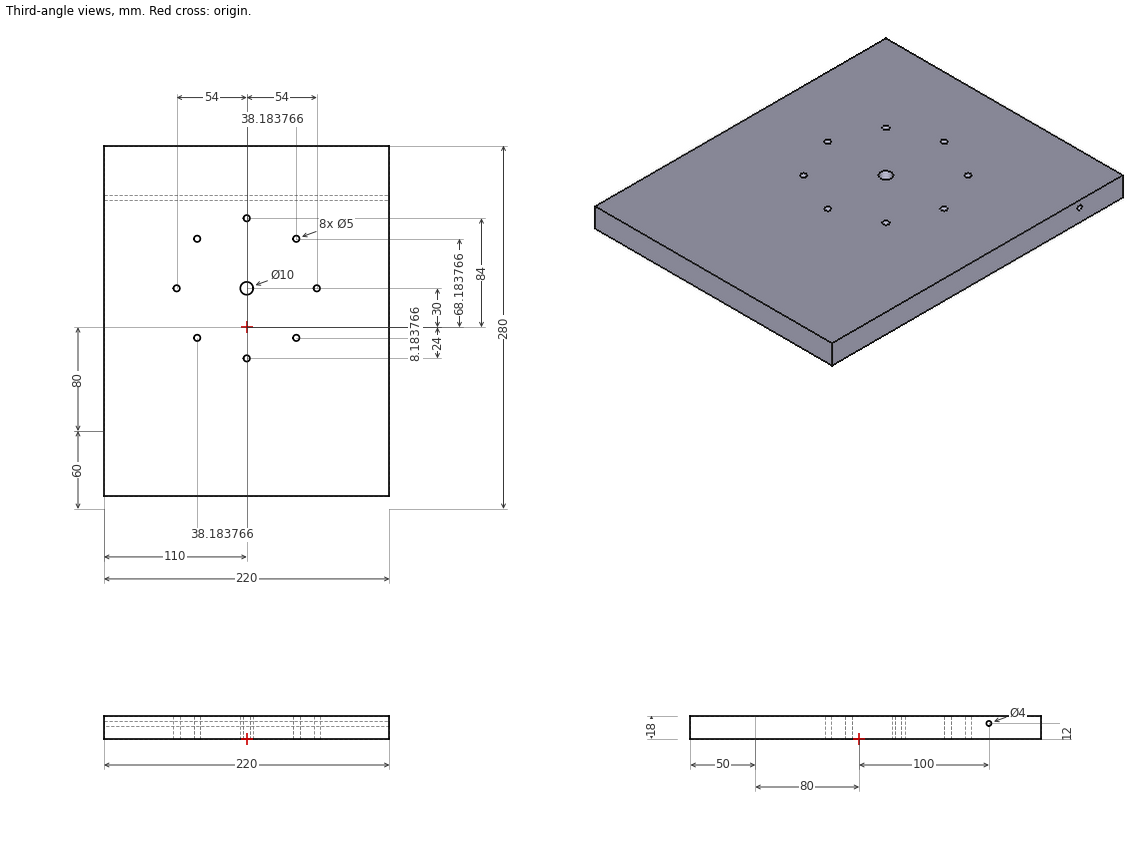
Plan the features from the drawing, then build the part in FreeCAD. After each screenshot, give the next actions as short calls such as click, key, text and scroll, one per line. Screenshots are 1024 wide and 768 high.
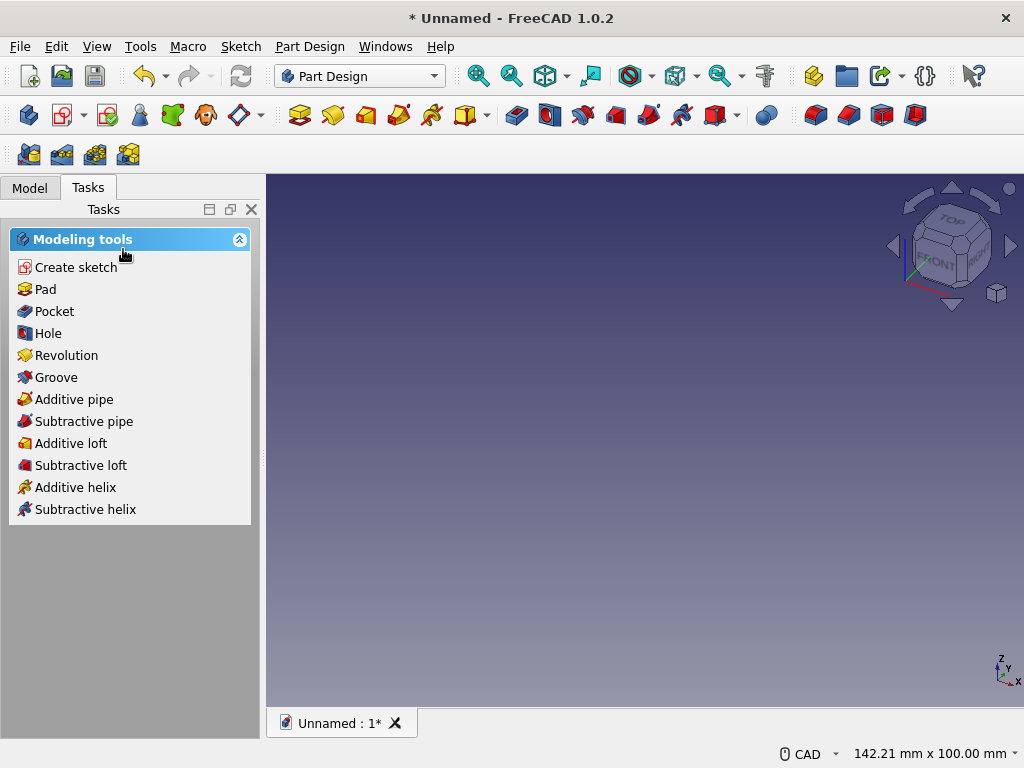
click(300, 116)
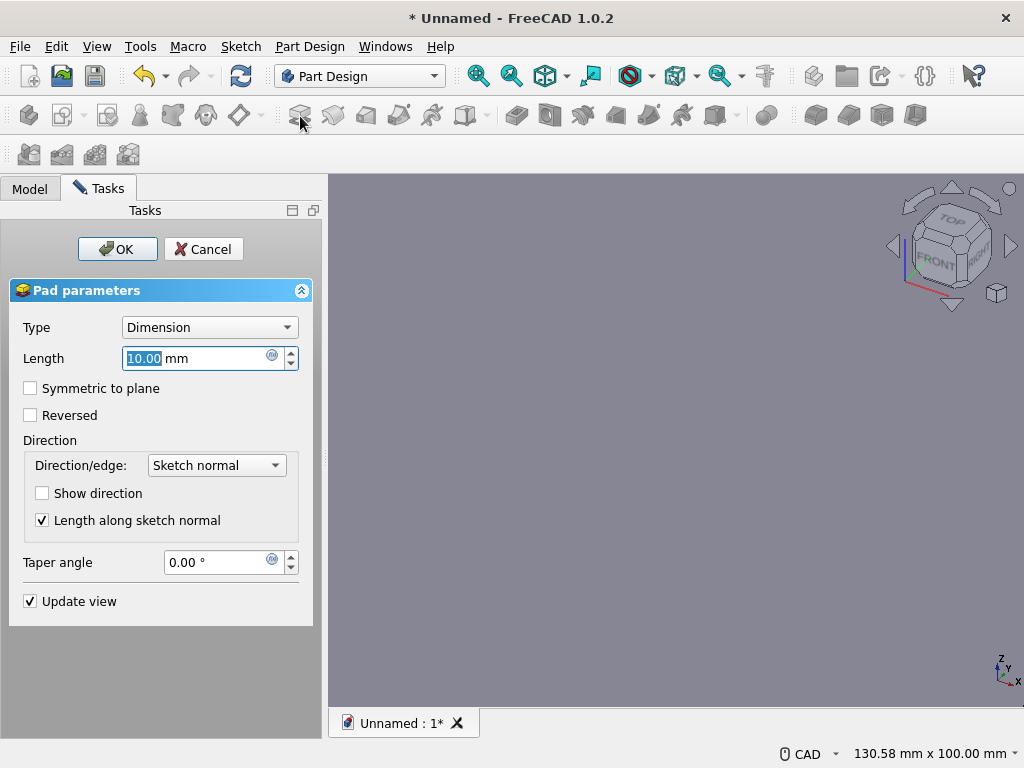
text(18)
key(Tab)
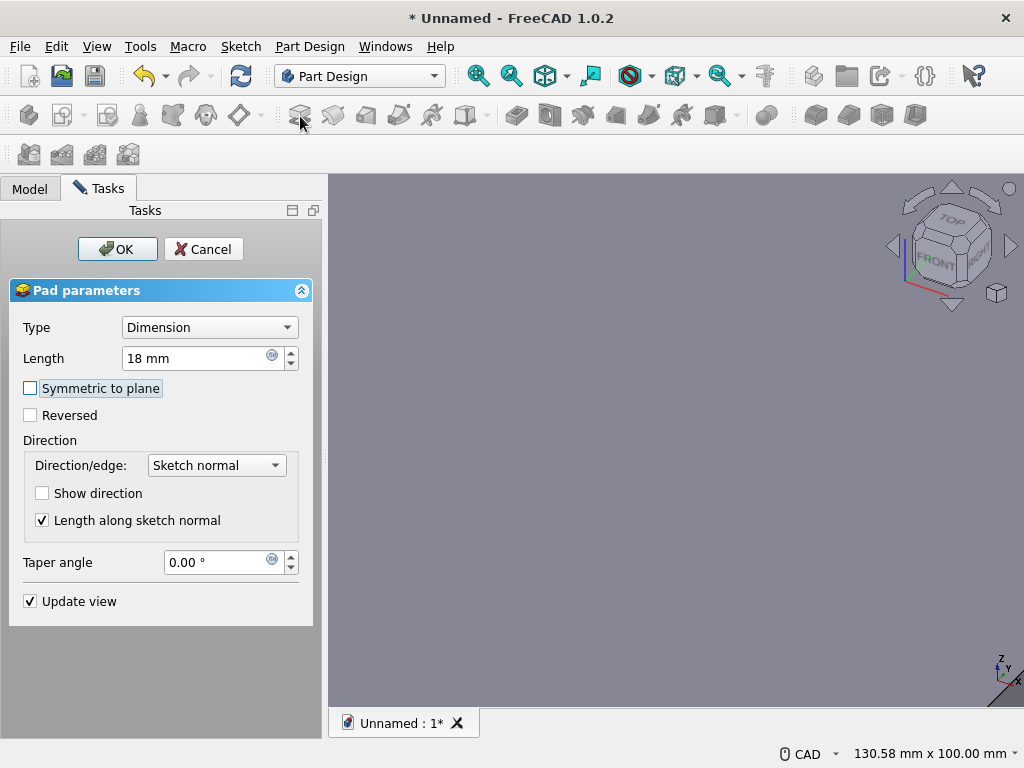
click(118, 249)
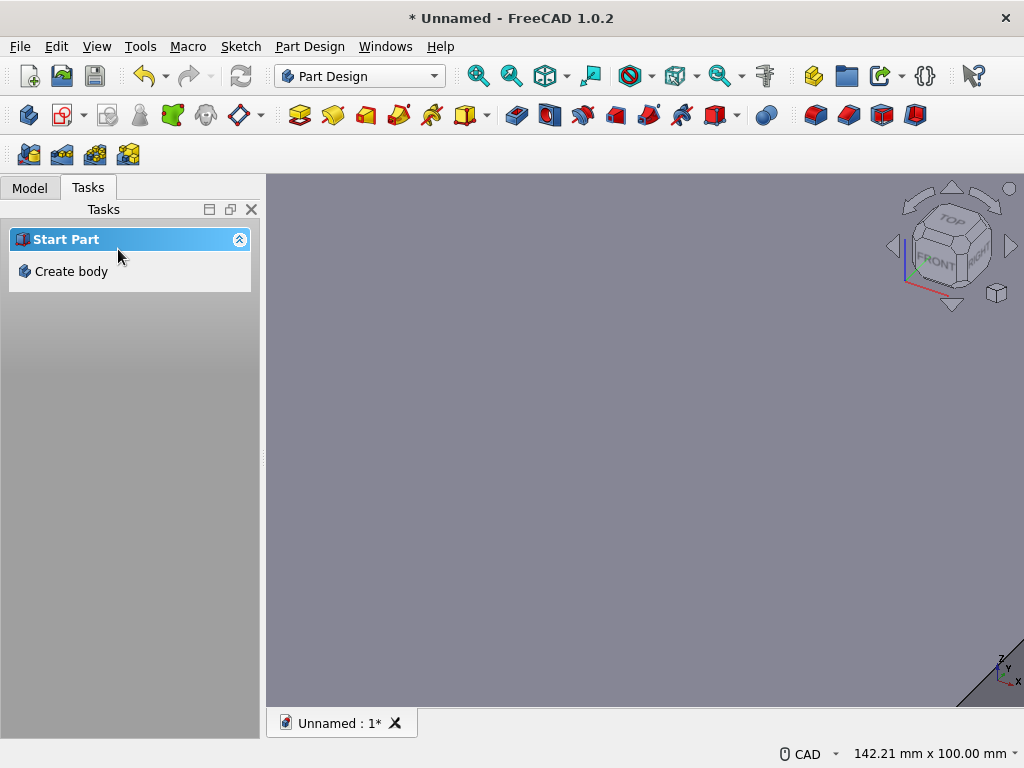
click(479, 76)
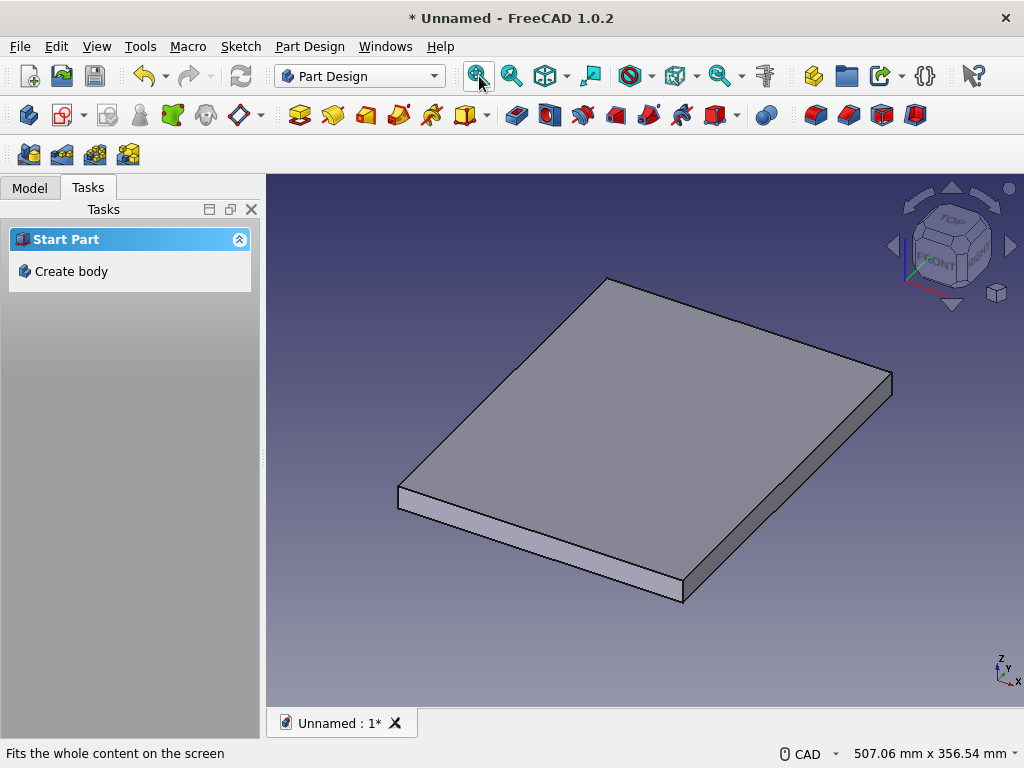
click(62, 116)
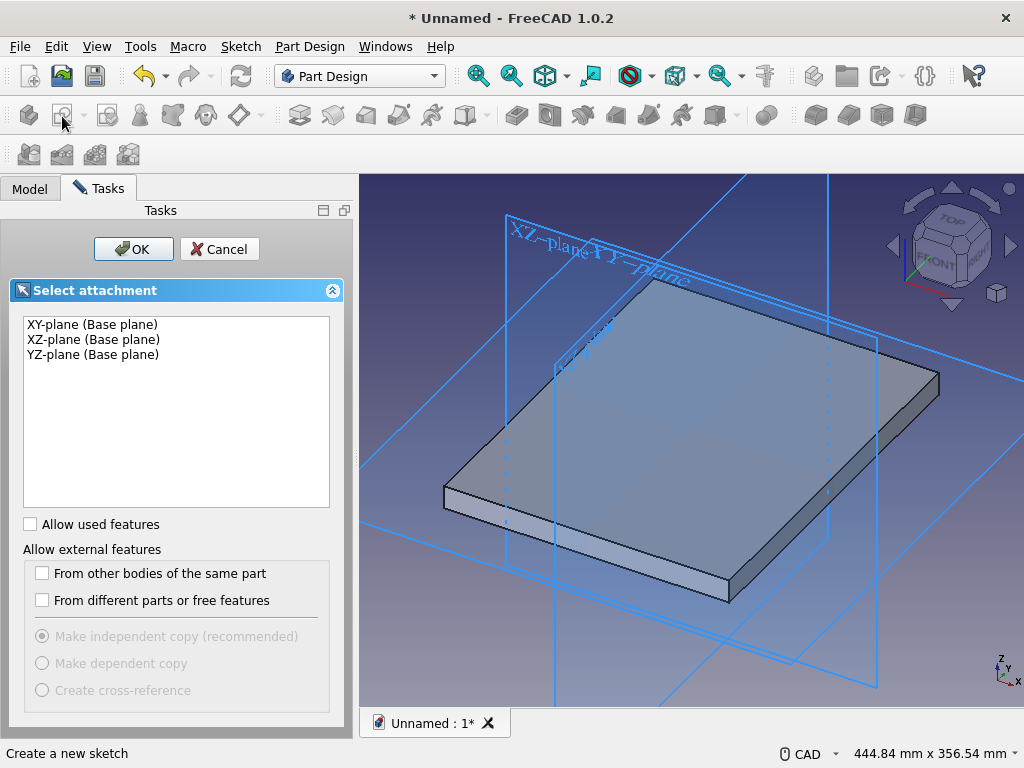
click(84, 324)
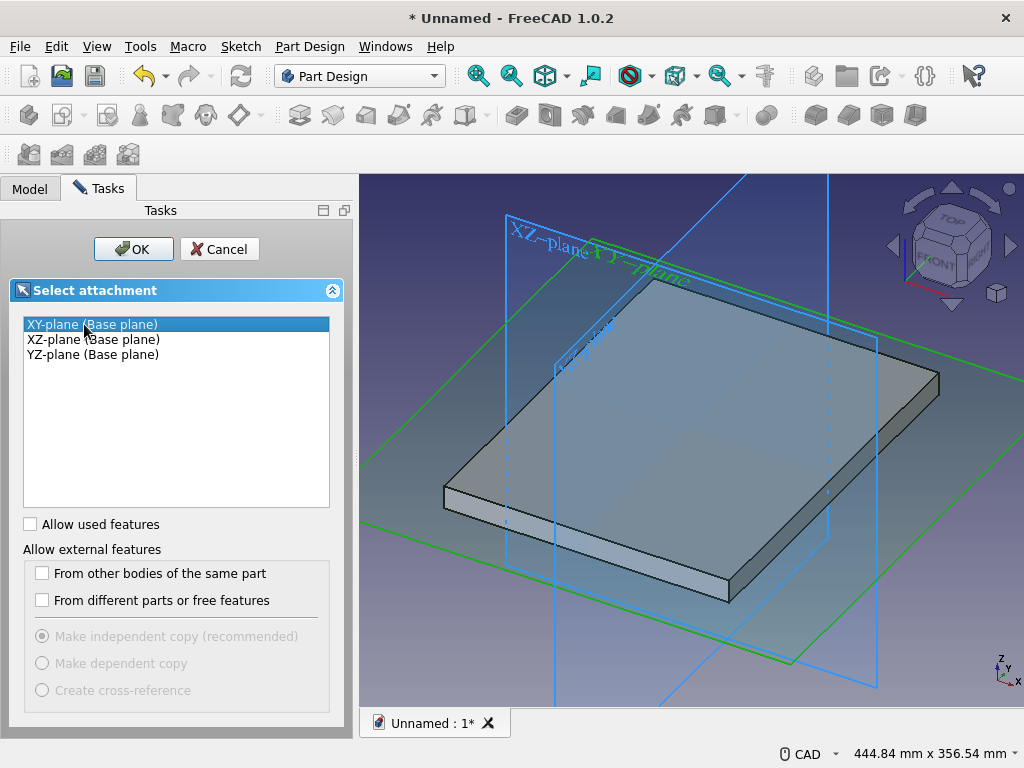
click(134, 249)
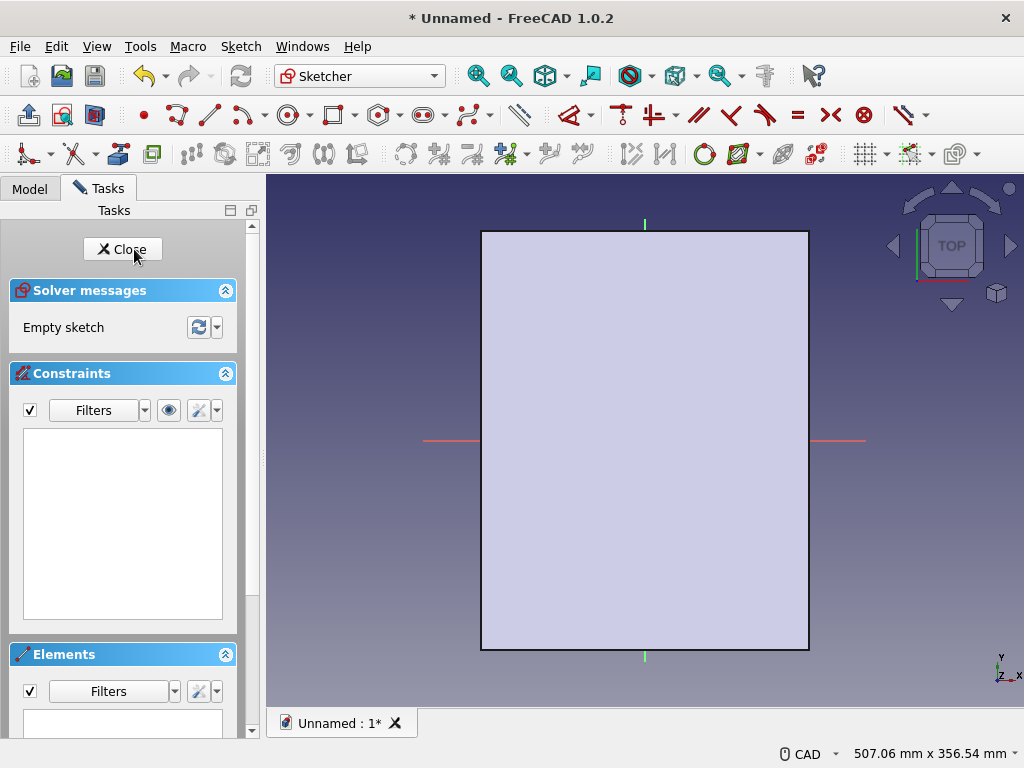
key(q)
key(s)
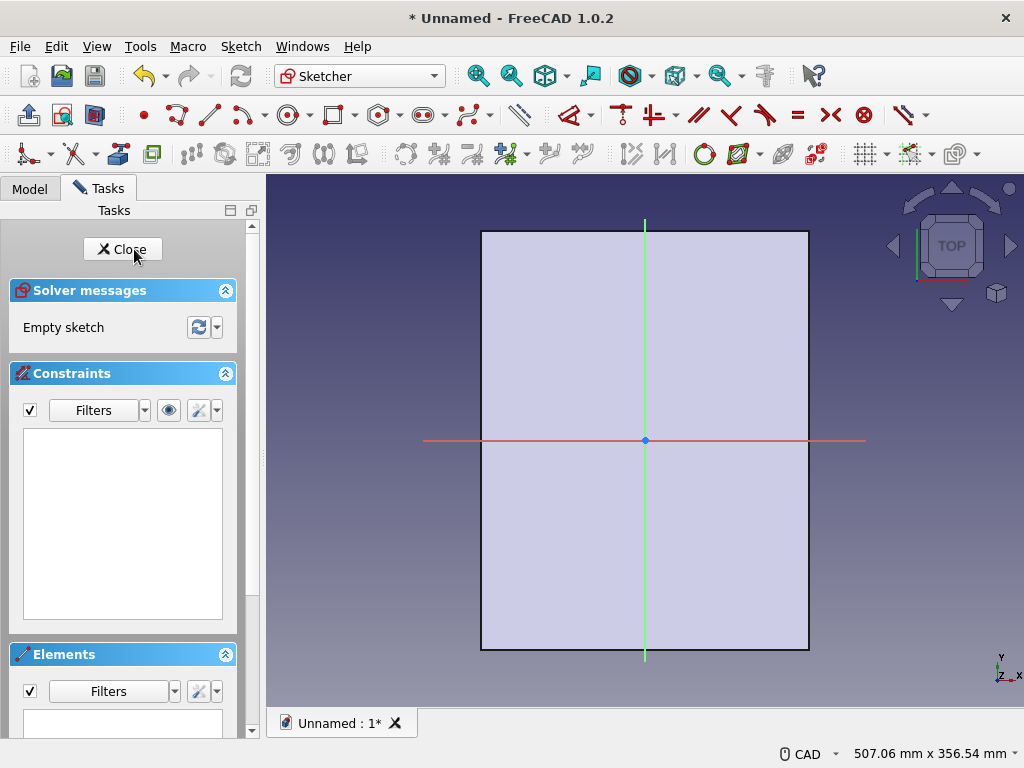
key(g)
key(r)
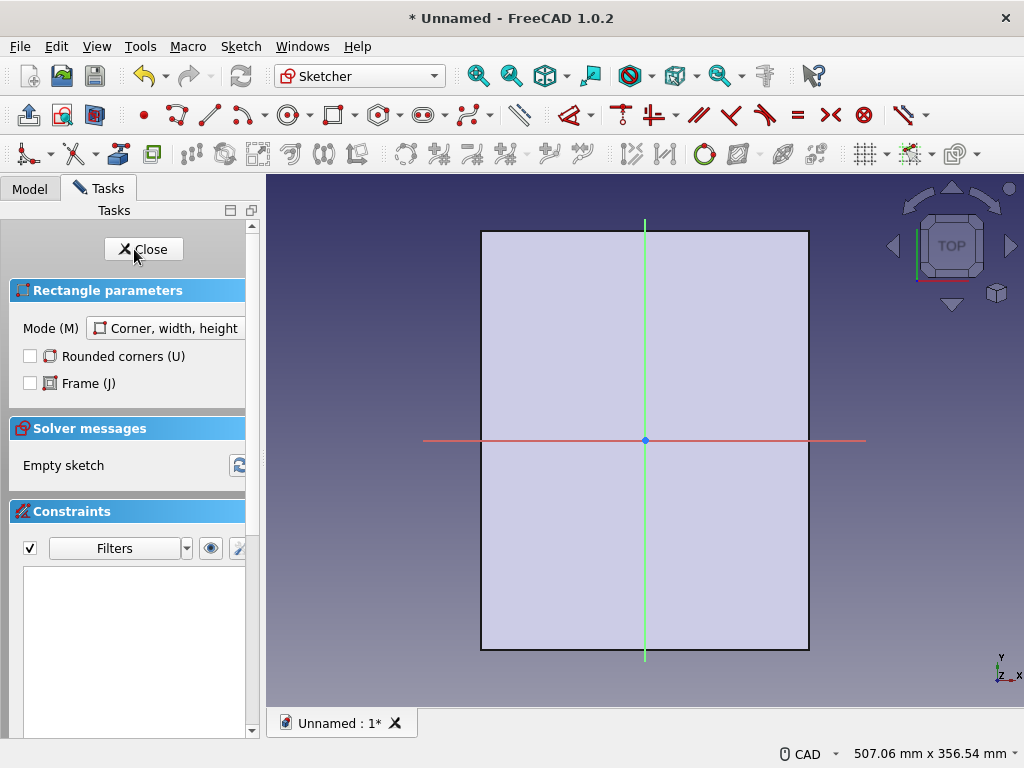
click(481, 560)
click(809, 650)
key(Escape)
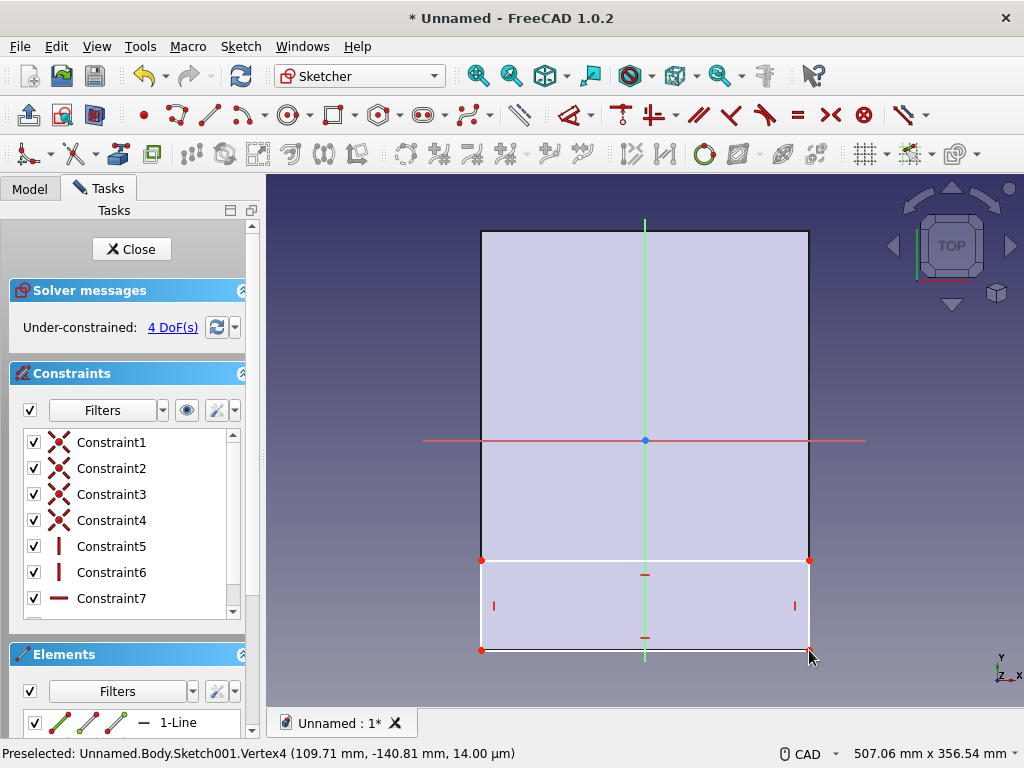
key(d)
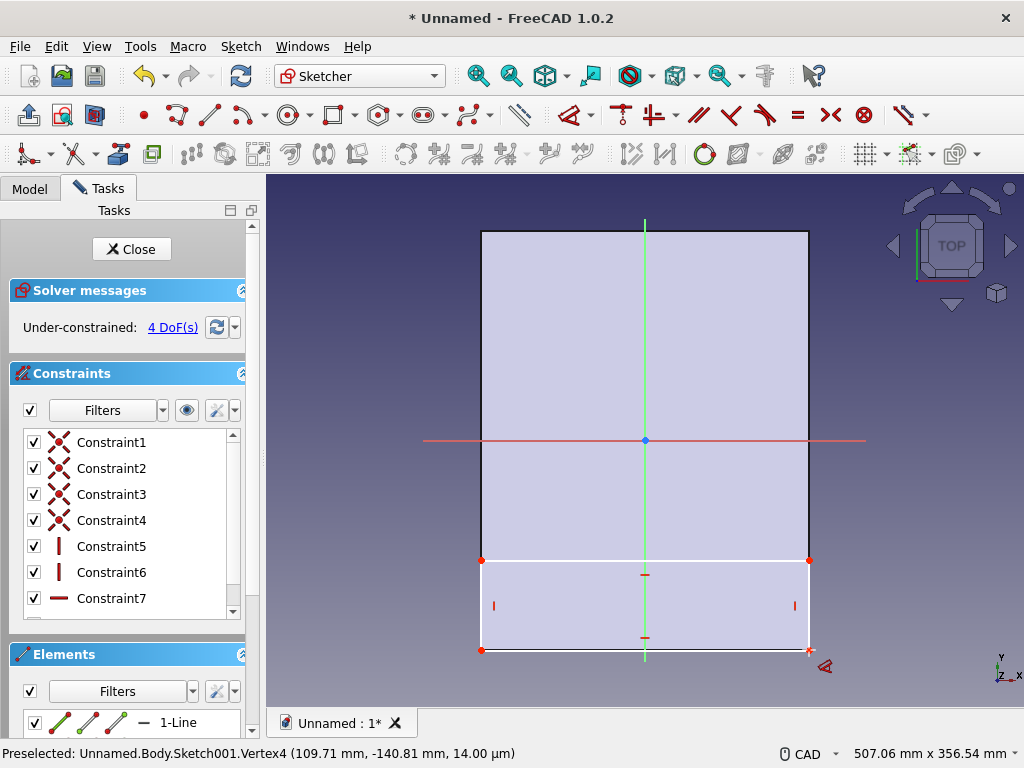
click(481, 588)
click(447, 606)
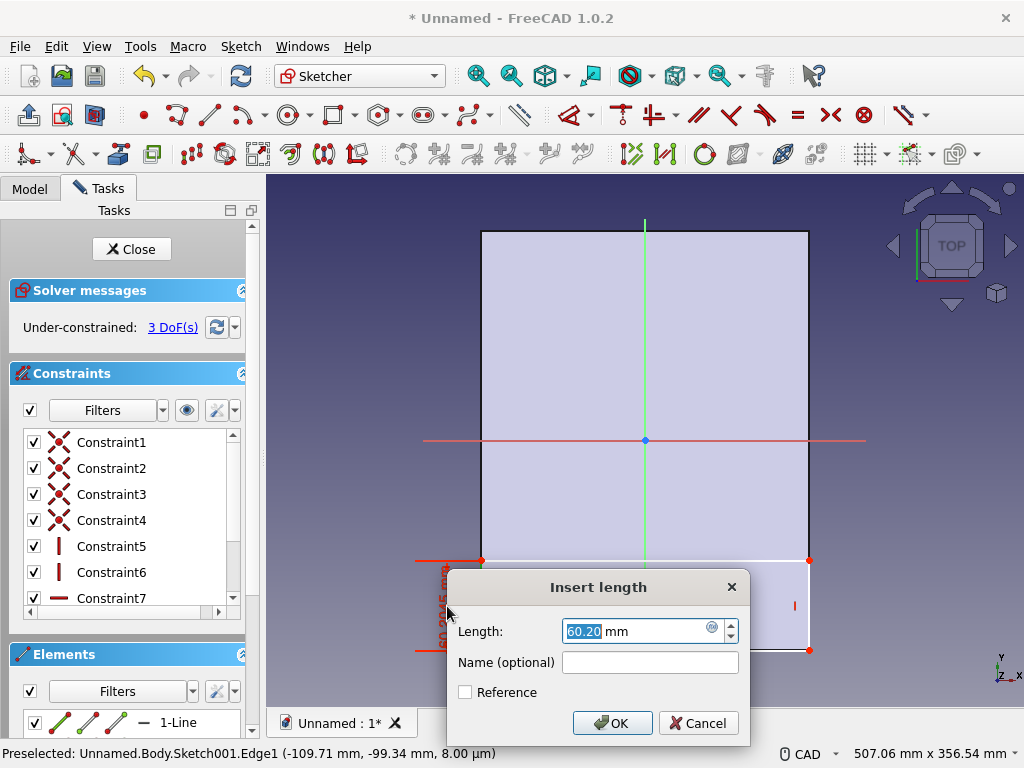
text(60)
key(Return)